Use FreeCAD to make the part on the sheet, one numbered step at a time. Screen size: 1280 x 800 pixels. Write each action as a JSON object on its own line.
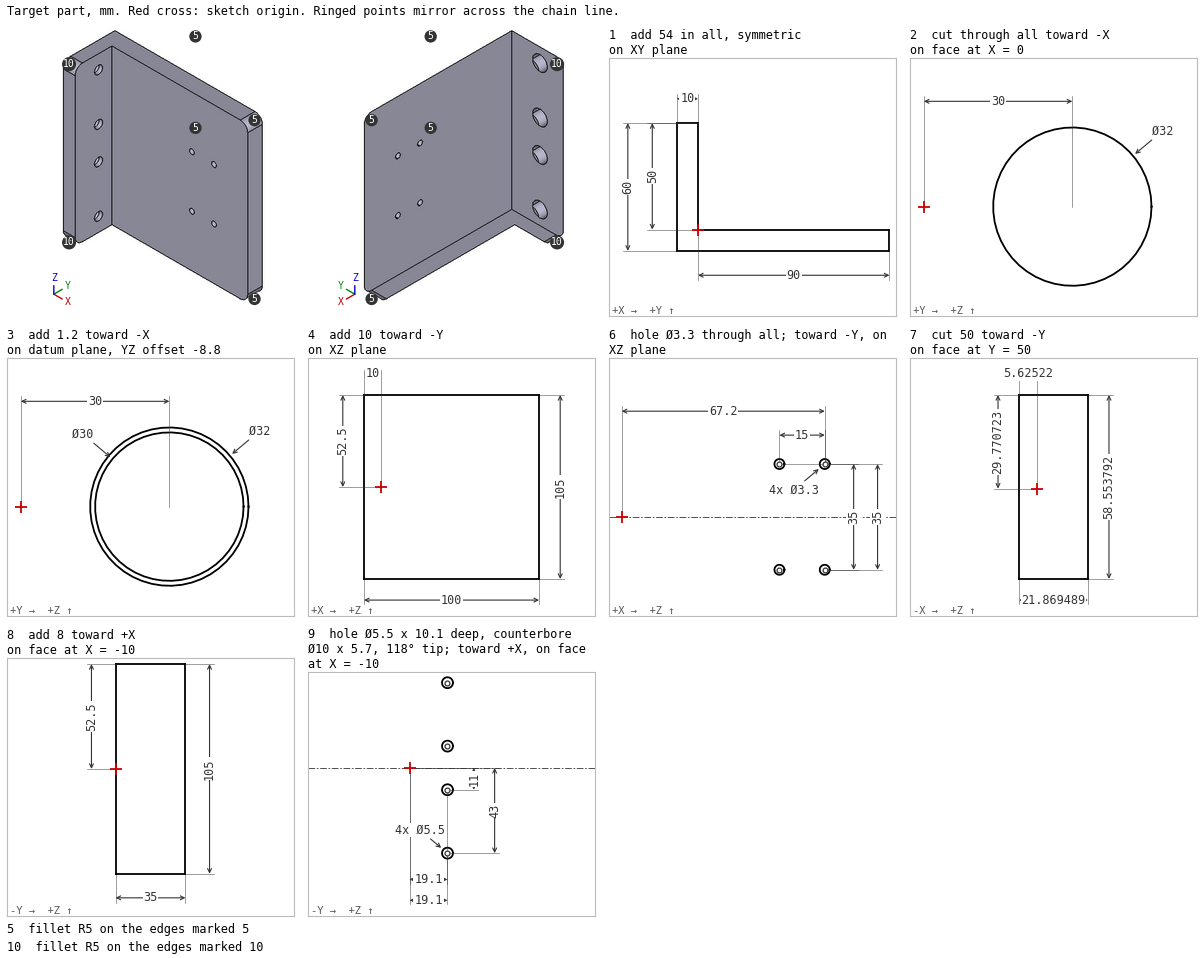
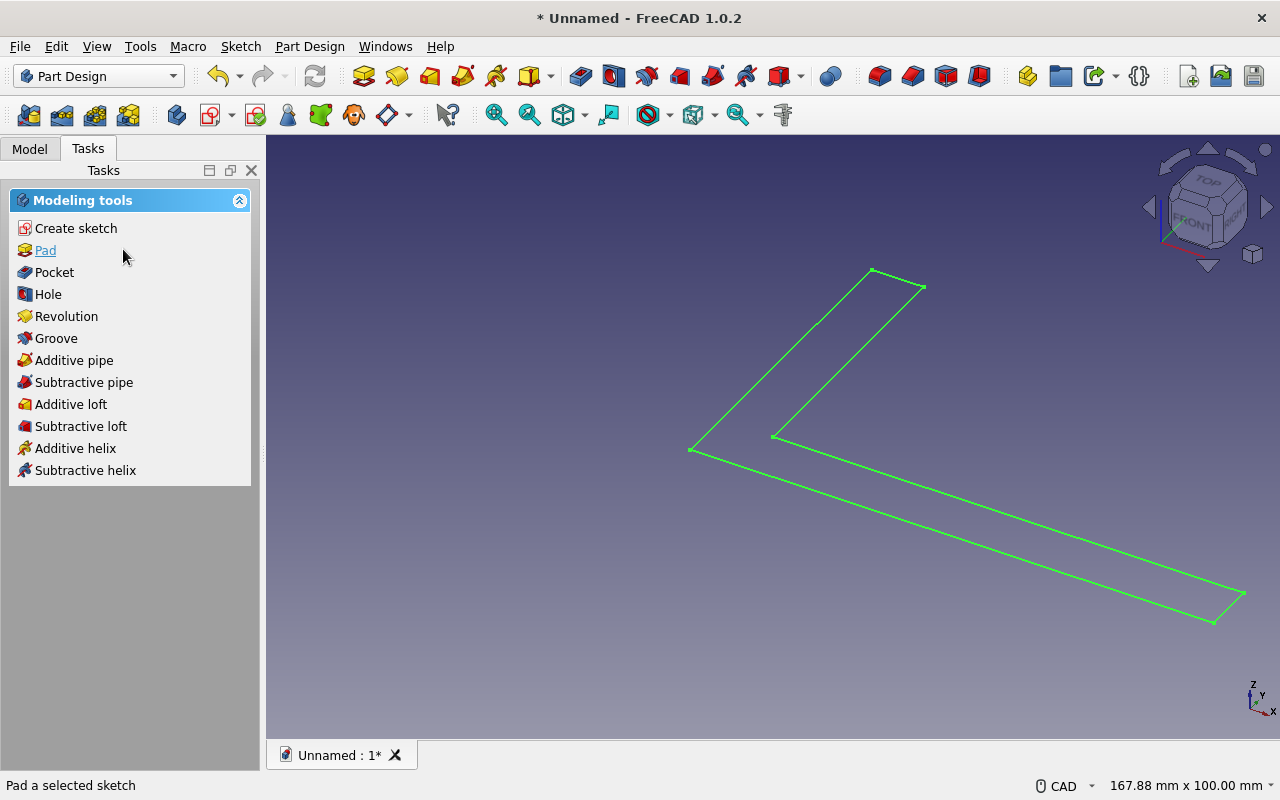
{"action": "left_click", "coordinate": [364, 76]}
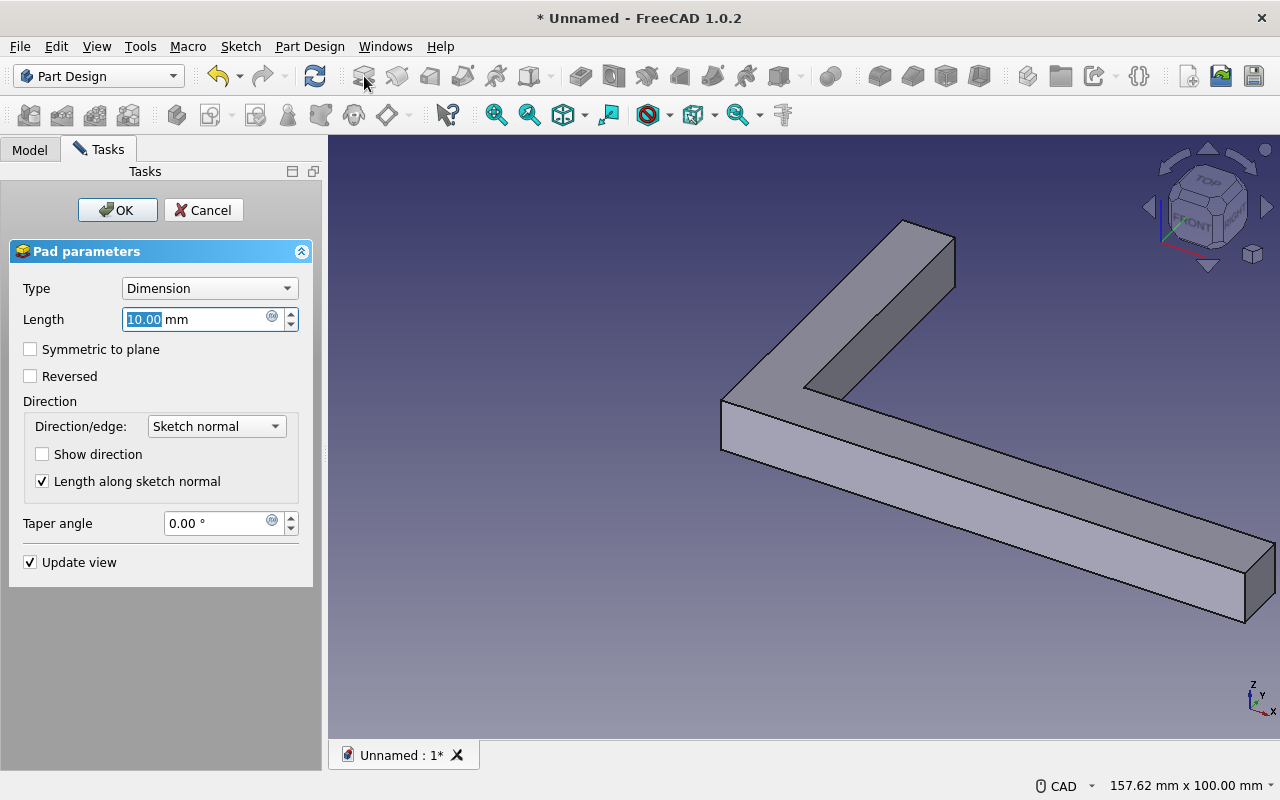
{"action": "type", "text": "54"}
{"action": "key", "text": "Tab"}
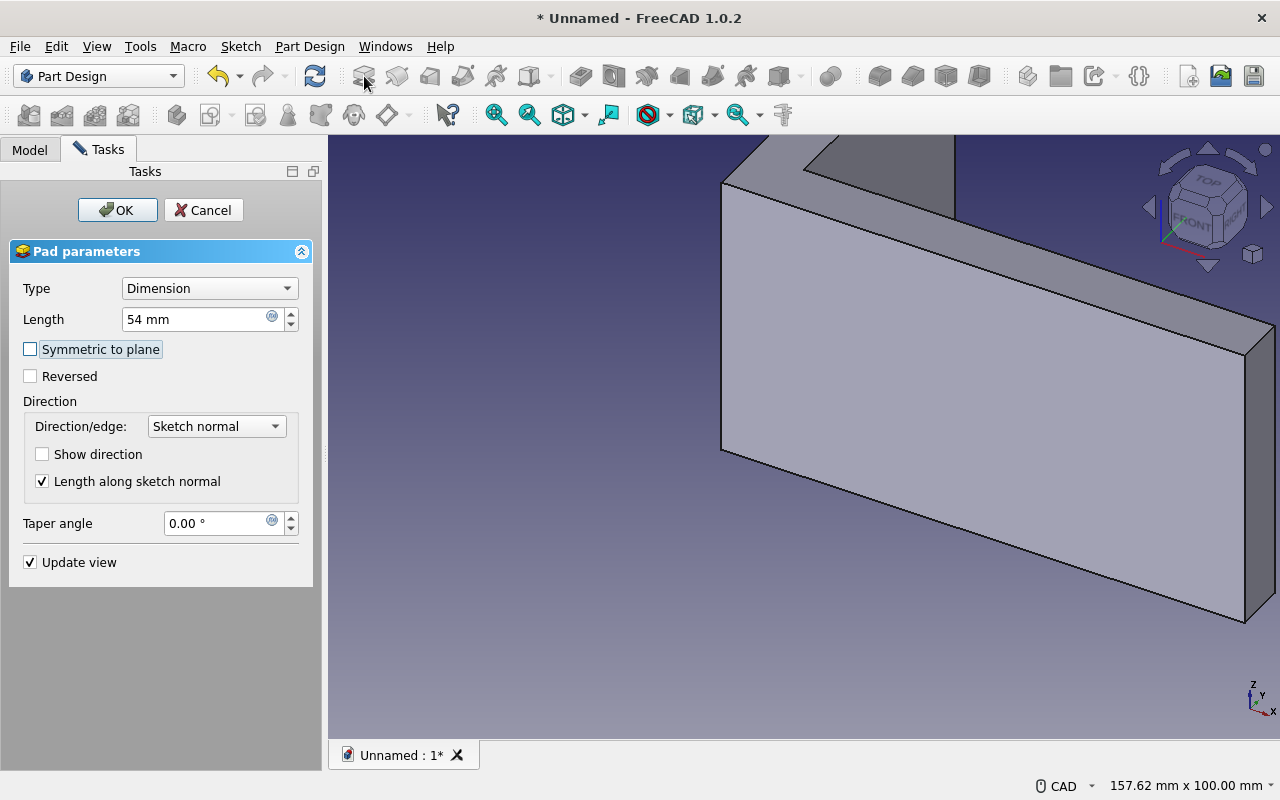
{"action": "left_click", "coordinate": [31, 349]}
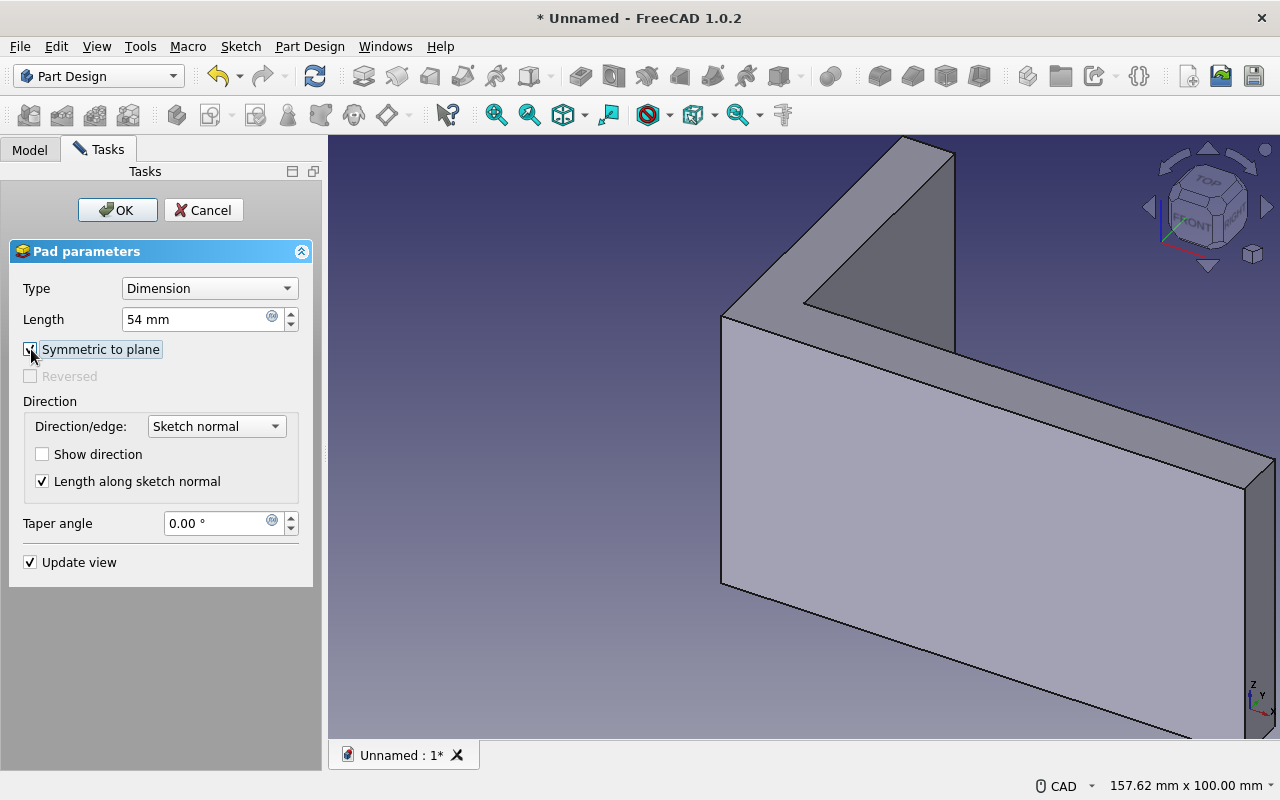
{"action": "left_click", "coordinate": [118, 210]}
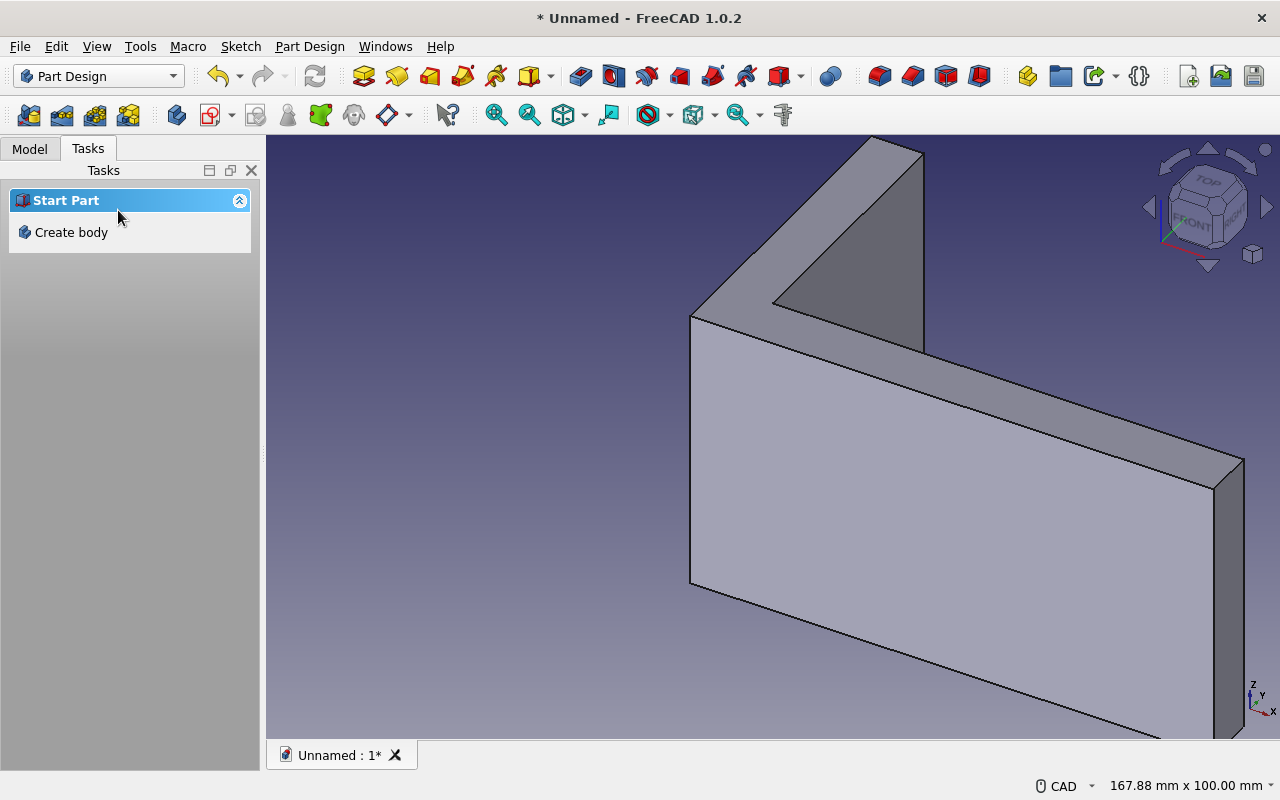
{"action": "left_click", "coordinate": [497, 116]}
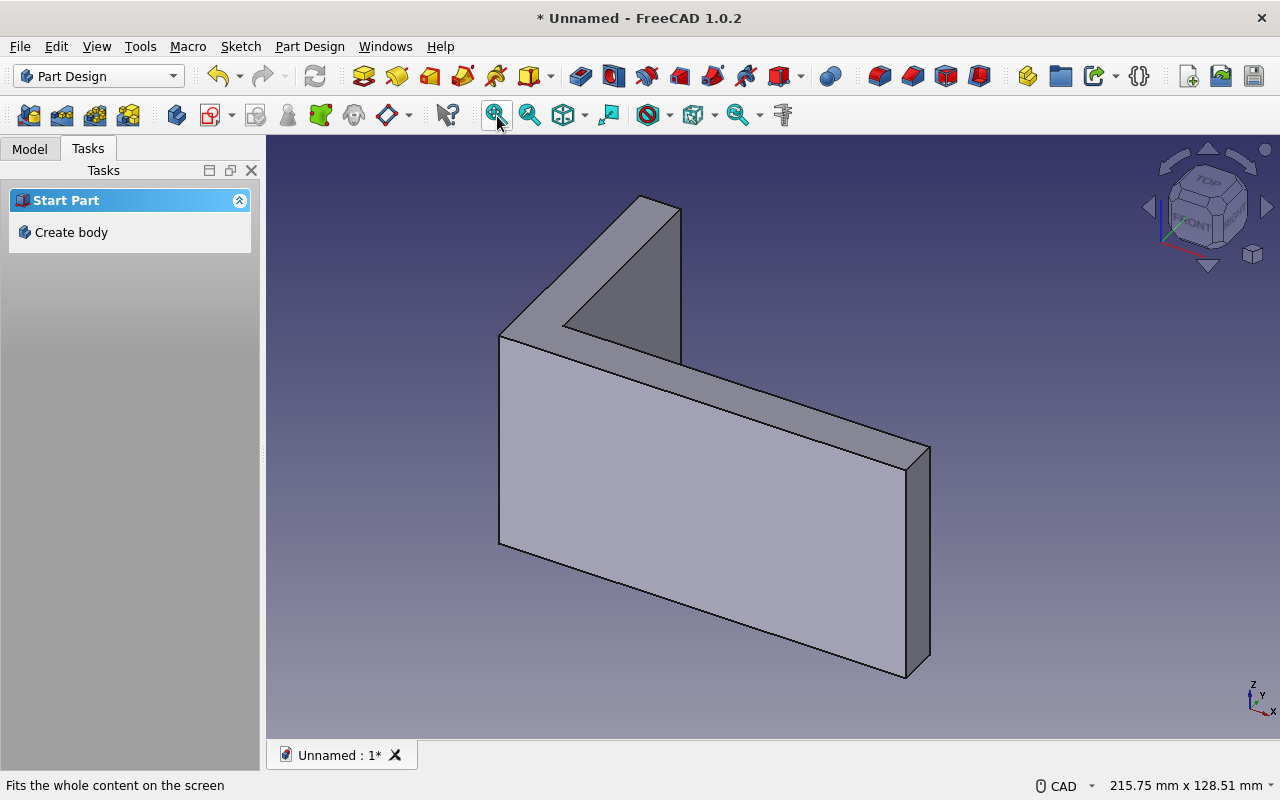
{"action": "left_click", "coordinate": [639, 324]}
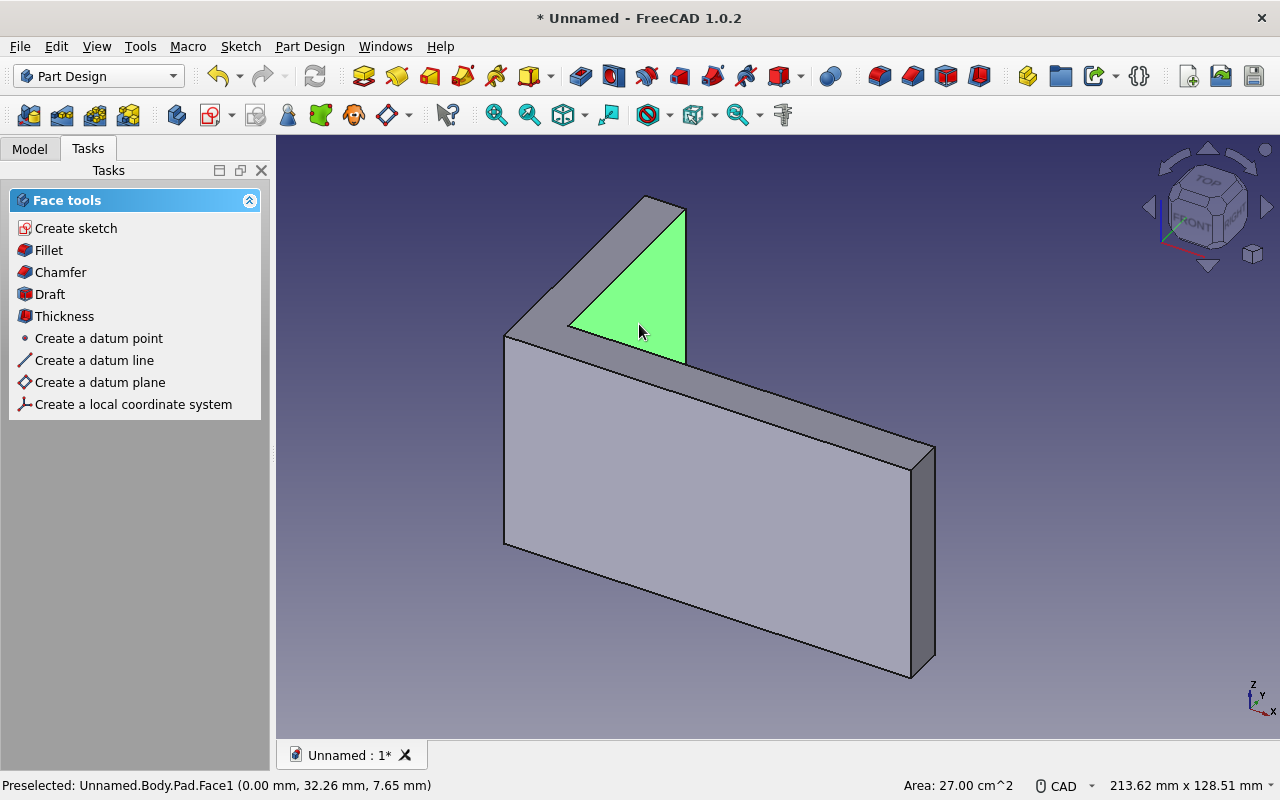
{"action": "left_click", "coordinate": [210, 116]}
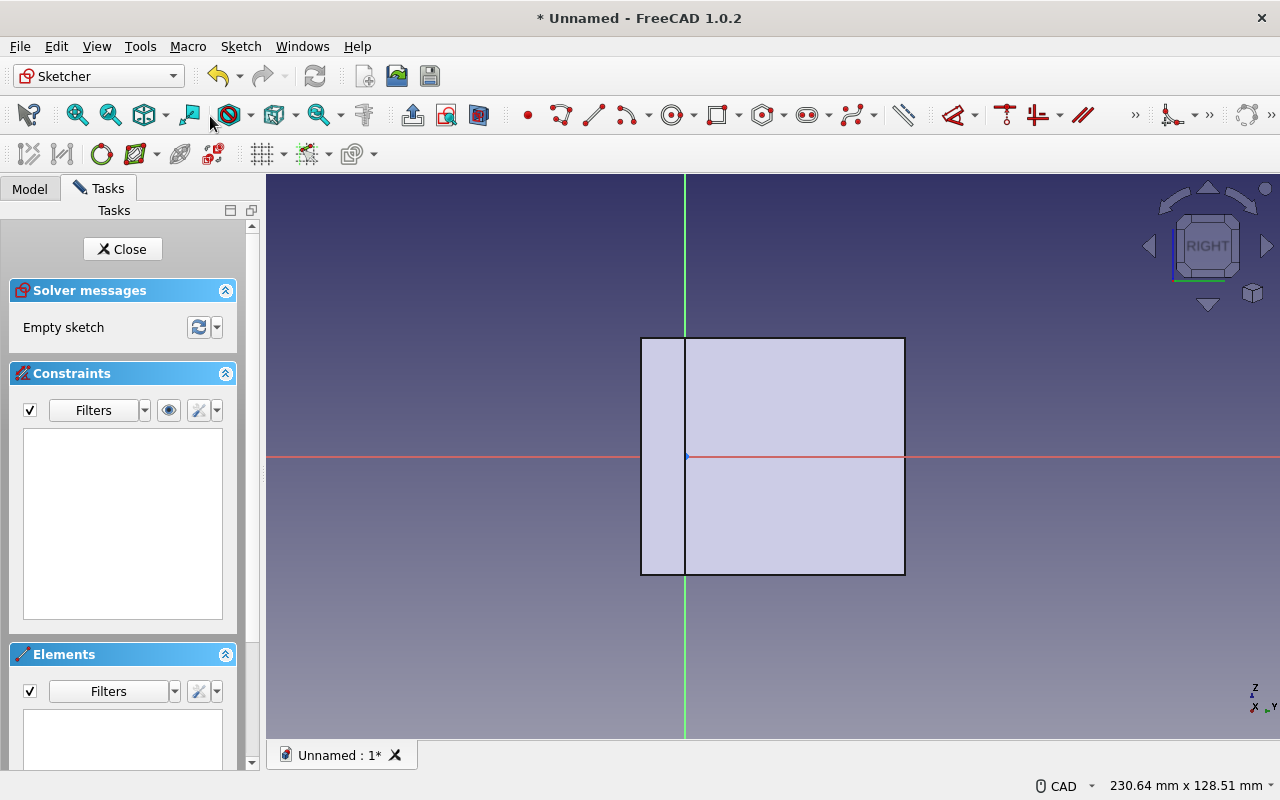
{"action": "left_click", "coordinate": [479, 116]}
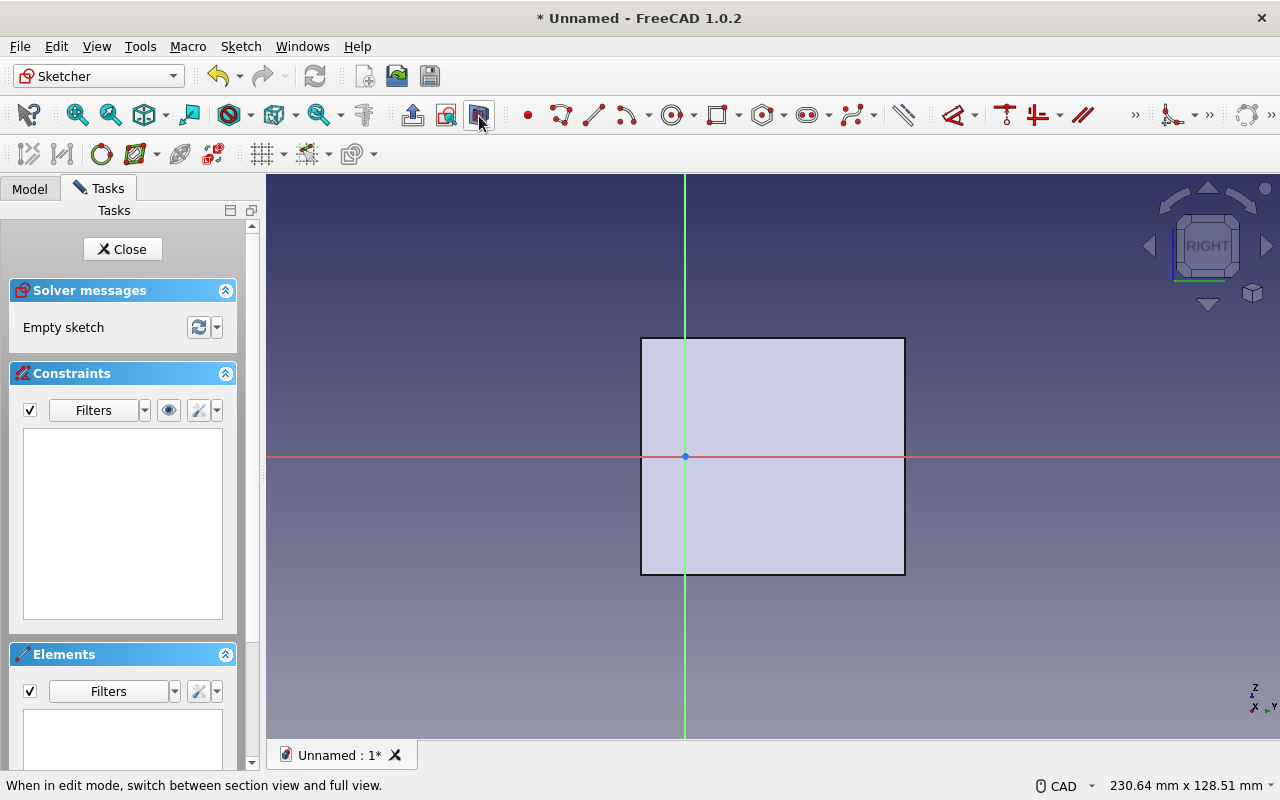
{"action": "scroll", "coordinate": [834, 456], "scroll_direction": "up", "scroll_amount": 5}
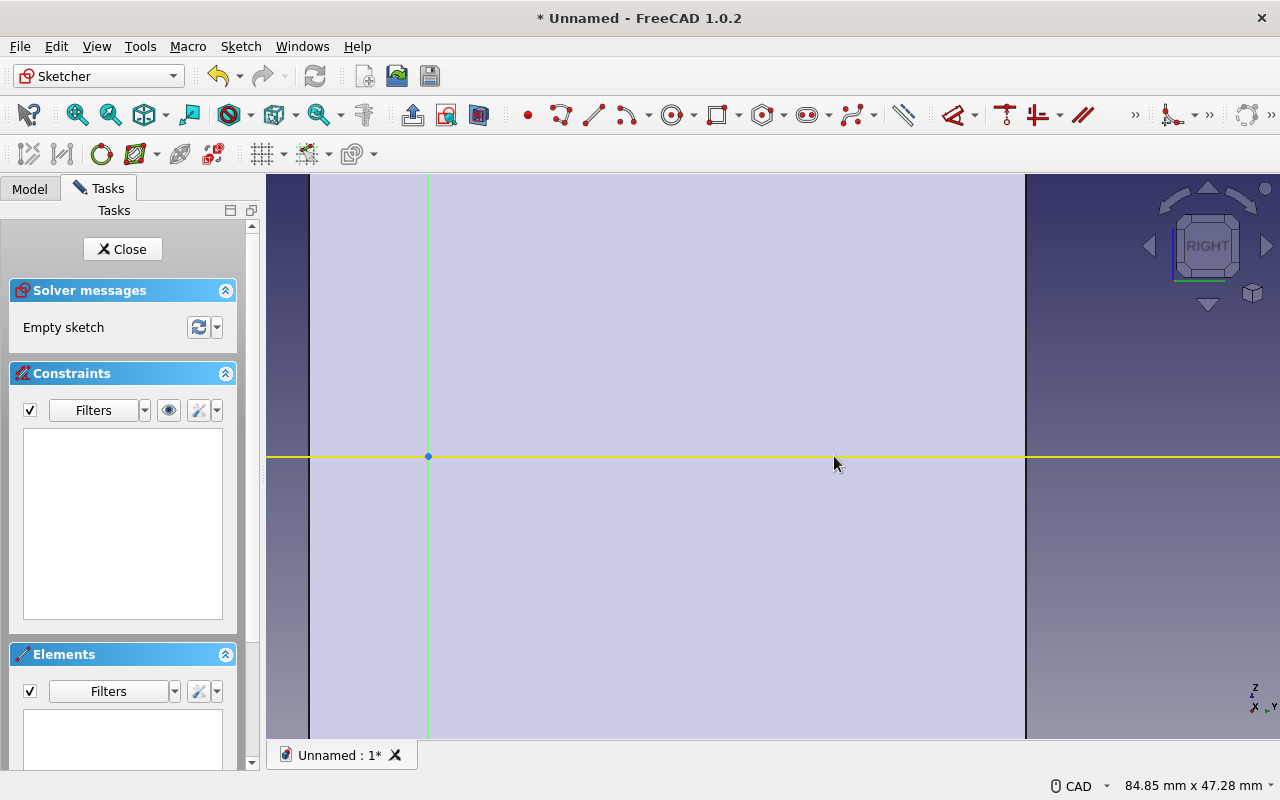
{"action": "left_click", "coordinate": [672, 116]}